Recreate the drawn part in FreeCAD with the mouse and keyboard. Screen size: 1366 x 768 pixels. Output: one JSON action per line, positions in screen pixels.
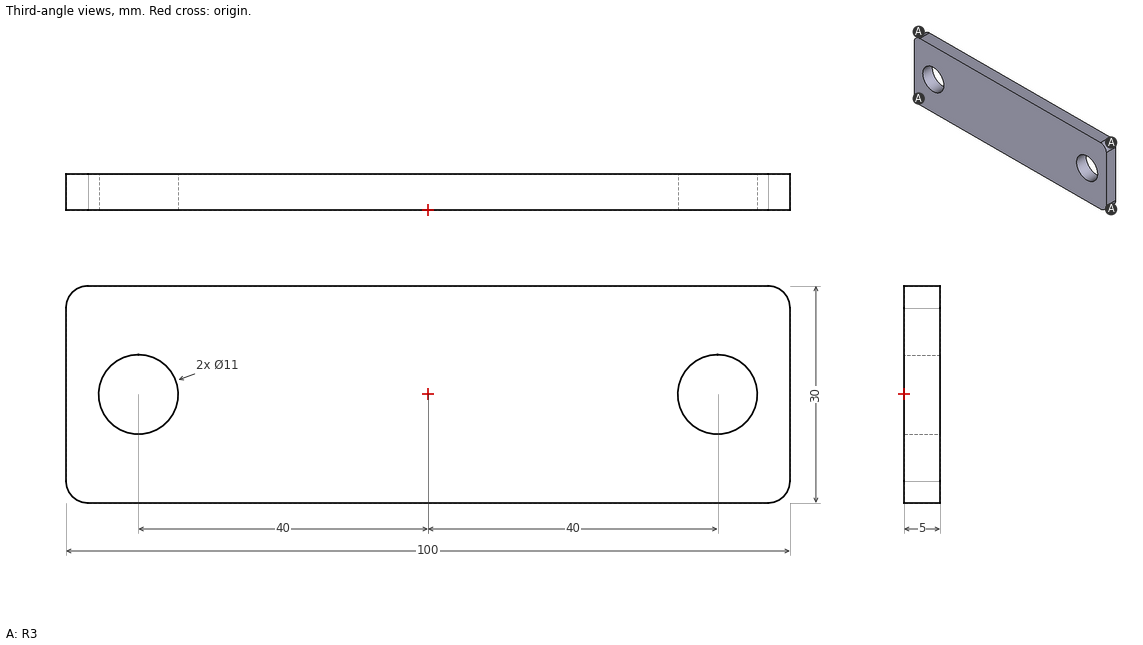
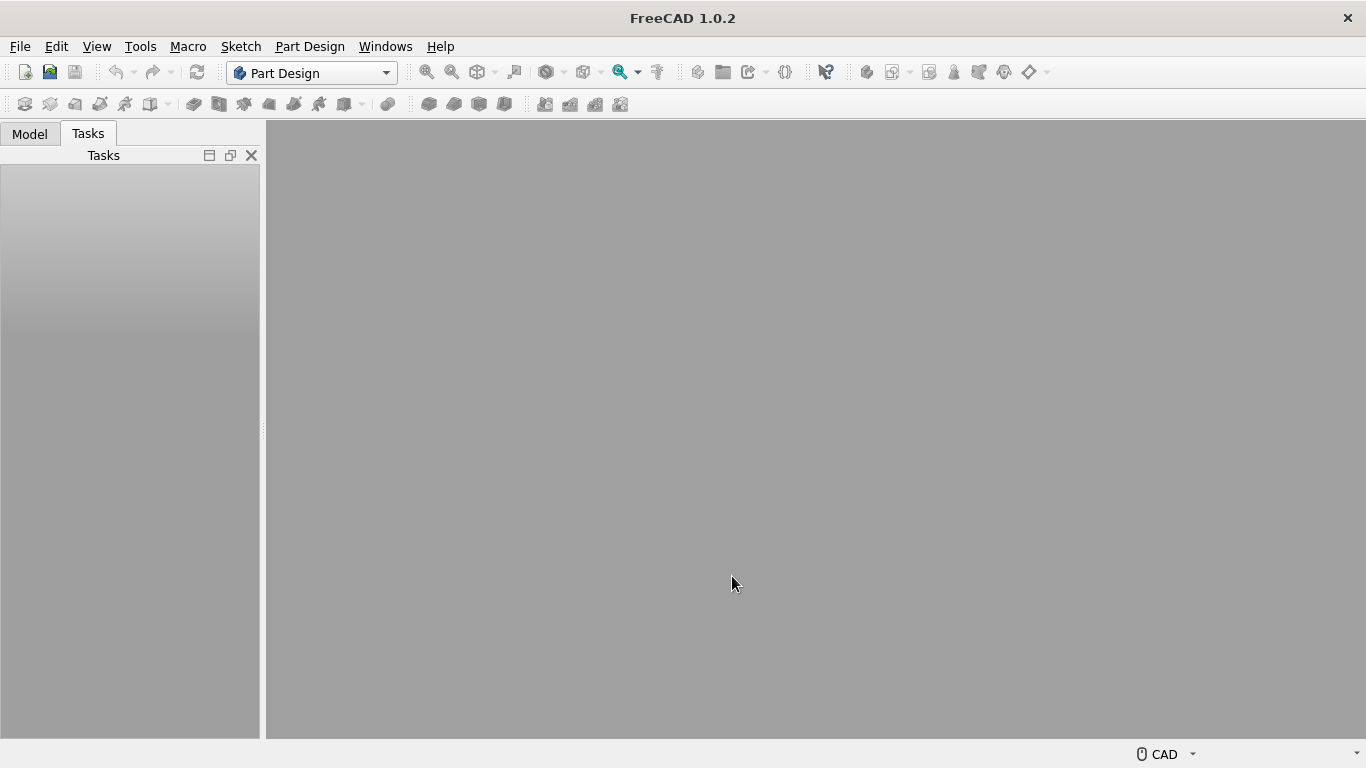
{"action": "key", "text": "ctrl+n"}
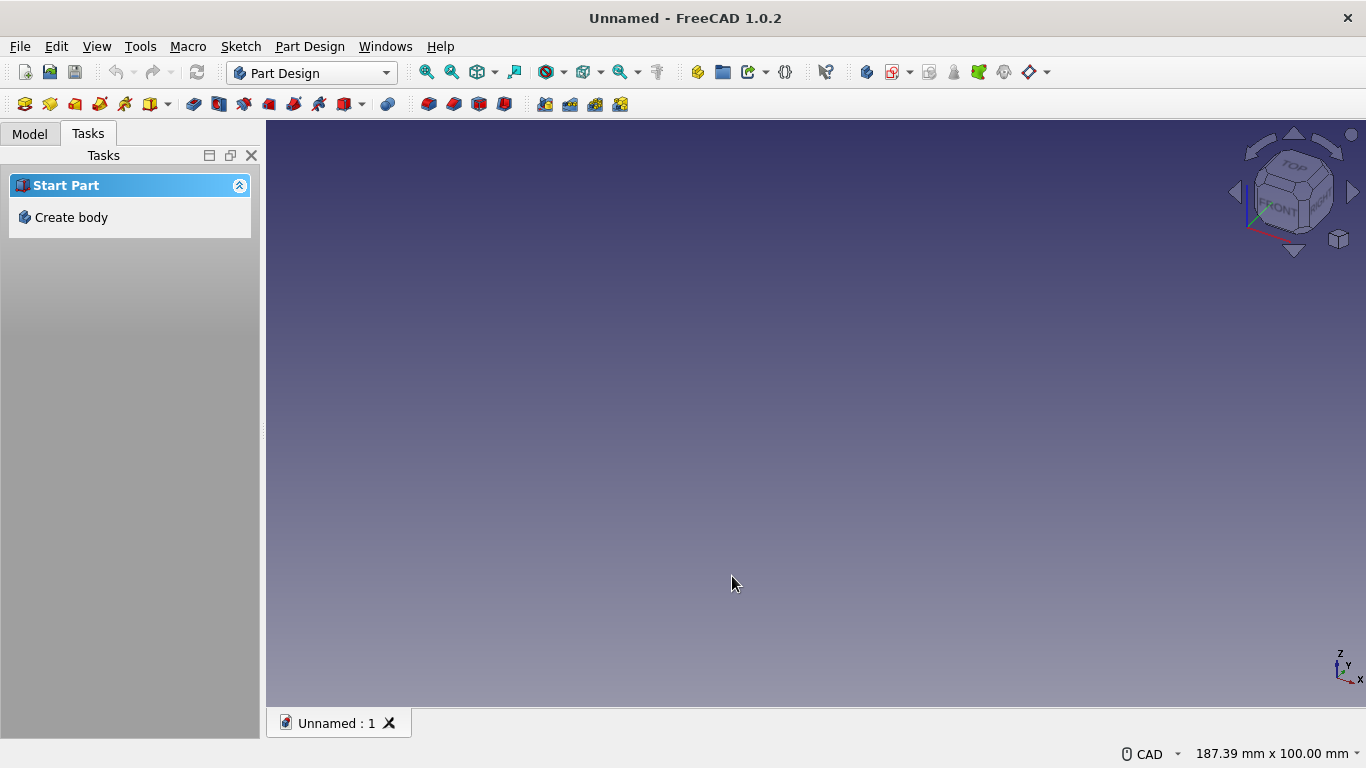
{"action": "left_click", "coordinate": [892, 72]}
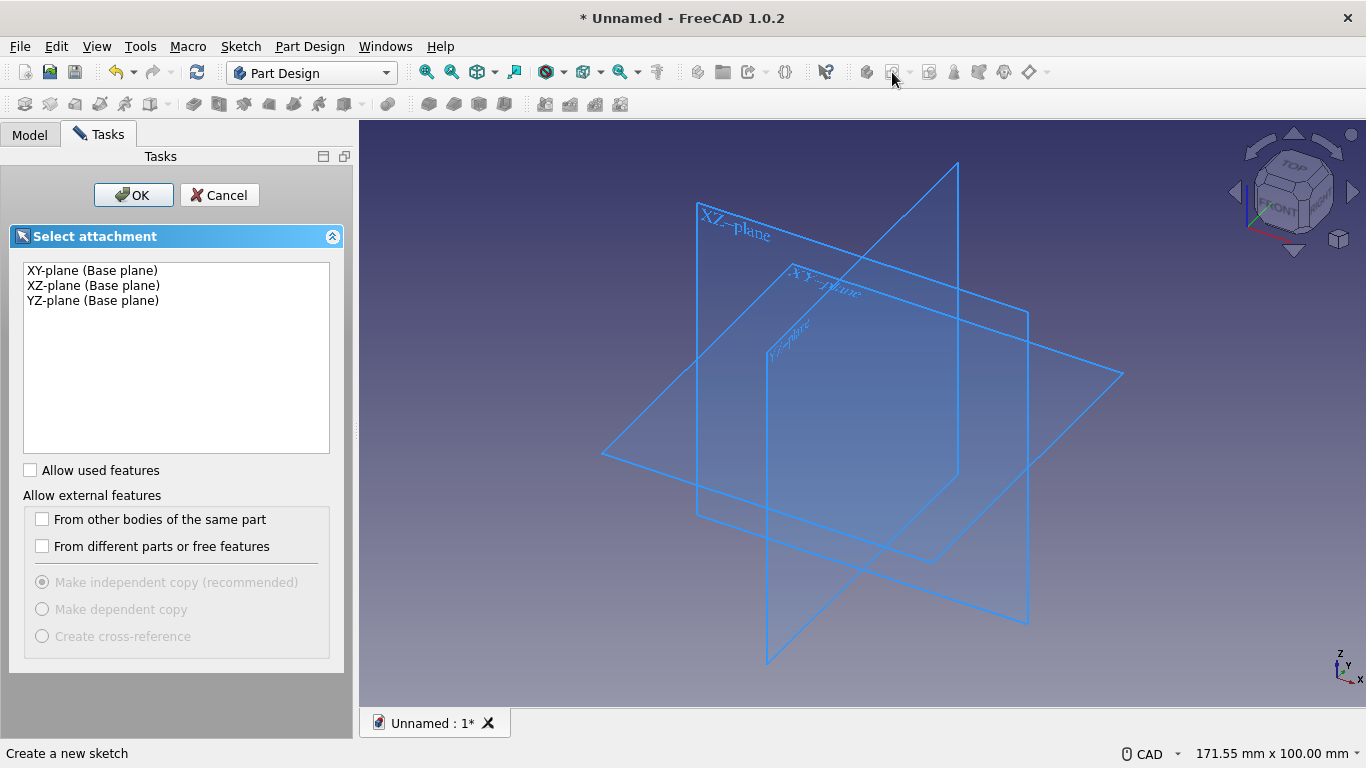
{"action": "left_click", "coordinate": [84, 286]}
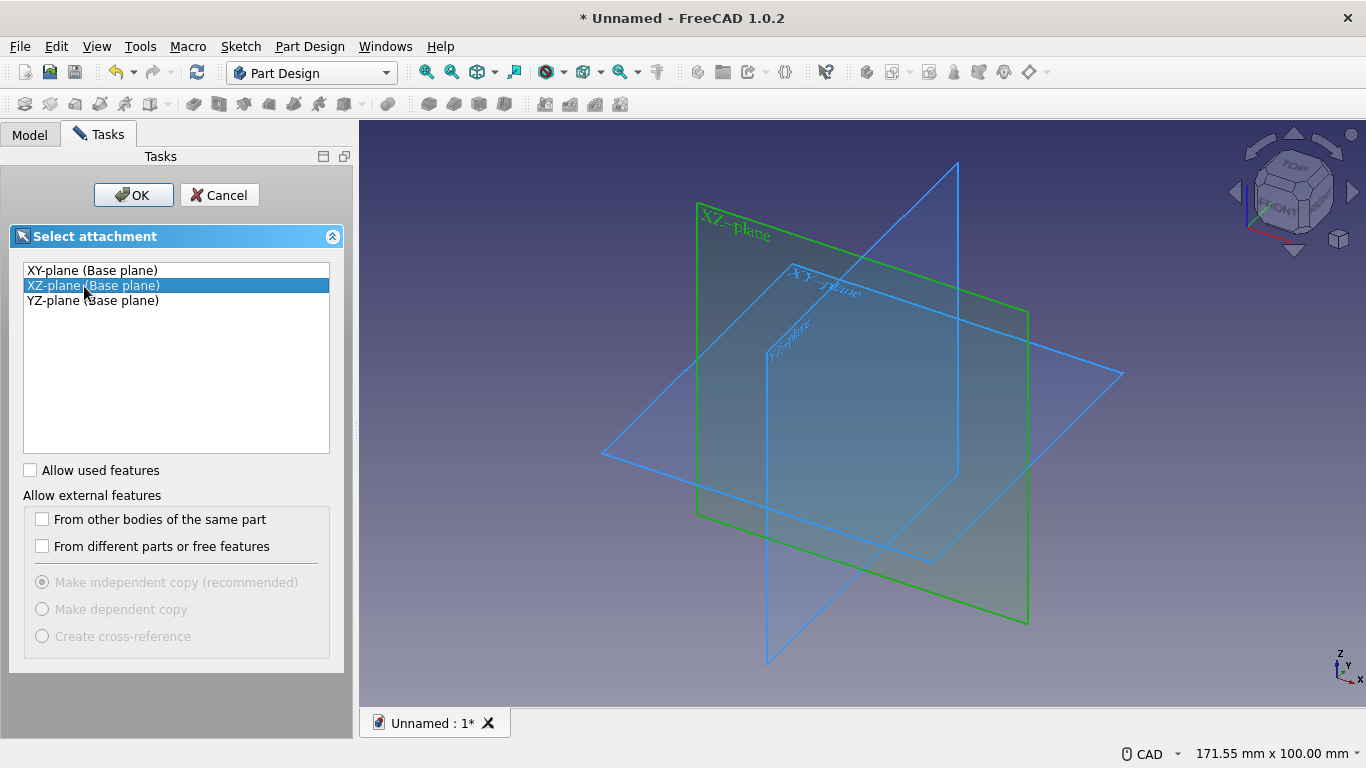
{"action": "left_click", "coordinate": [134, 195]}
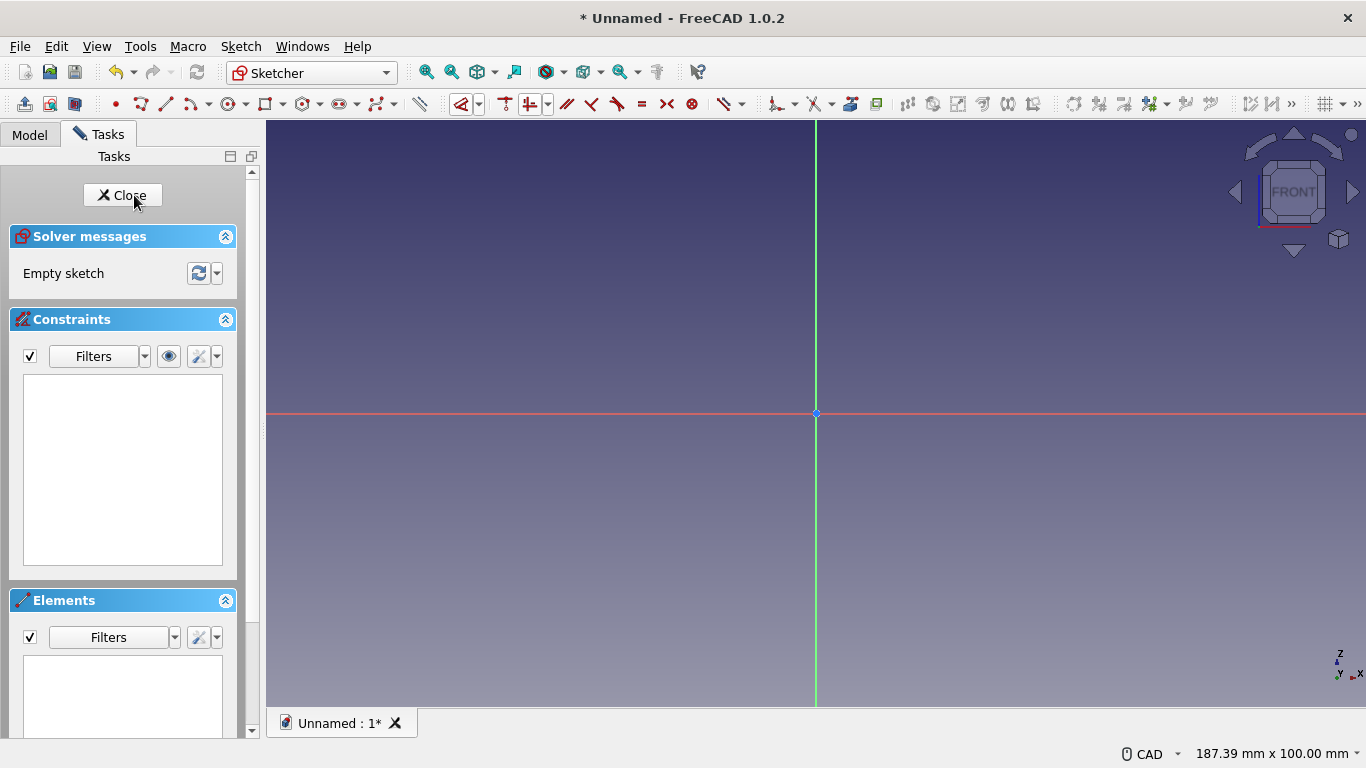
{"action": "key", "text": "g v"}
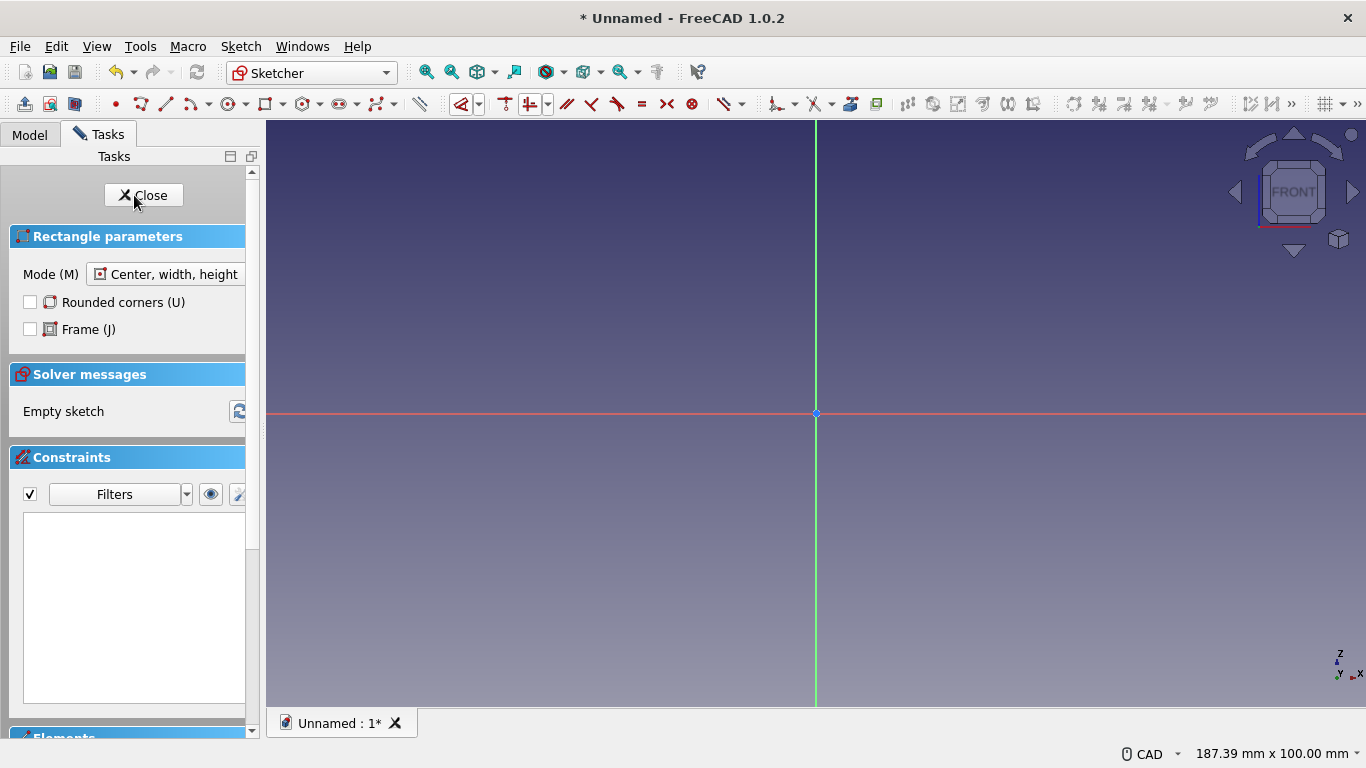
{"action": "left_click", "coordinate": [816, 414]}
{"action": "mouse_move", "coordinate": [1110, 325]}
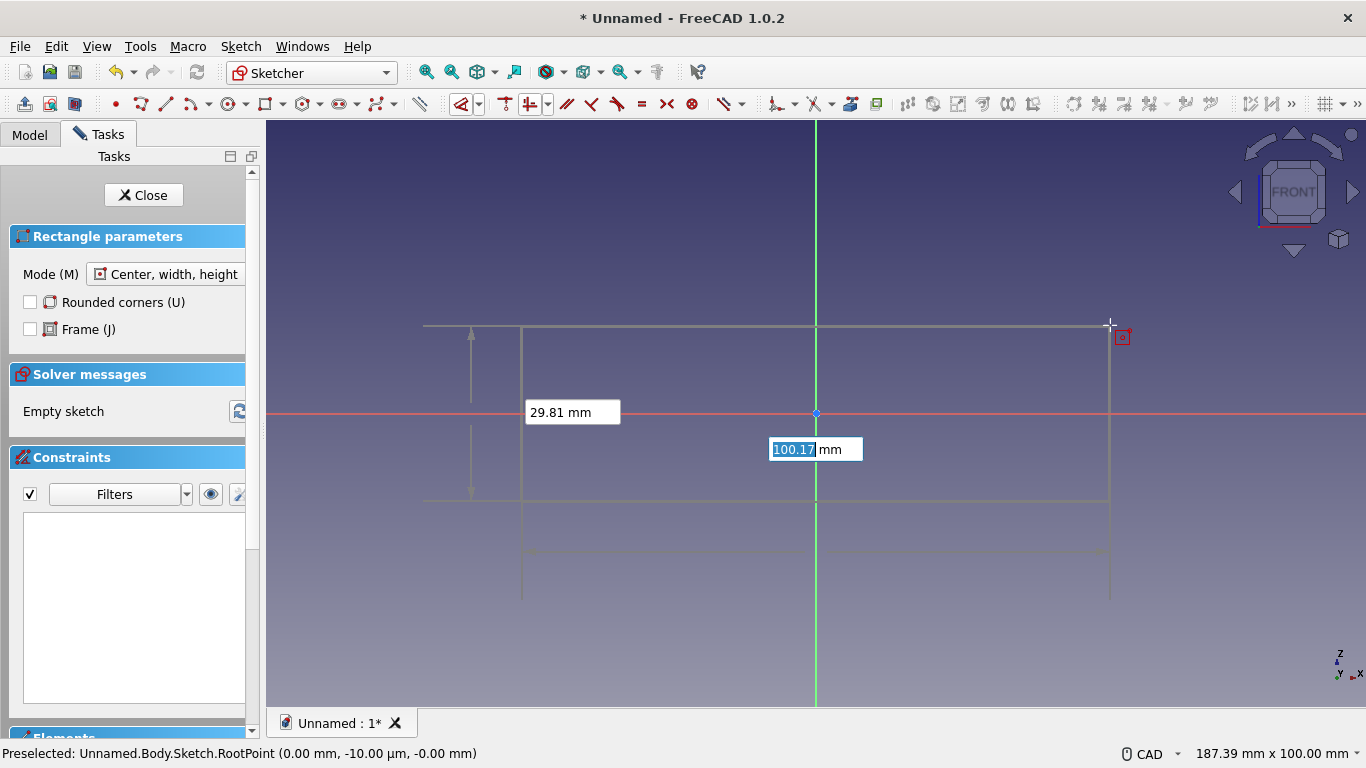
{"action": "type", "text": "100"}
{"action": "key", "text": "Tab"}
{"action": "type", "text": "30"}
{"action": "key", "text": "Return"}
{"action": "key", "text": "Escape"}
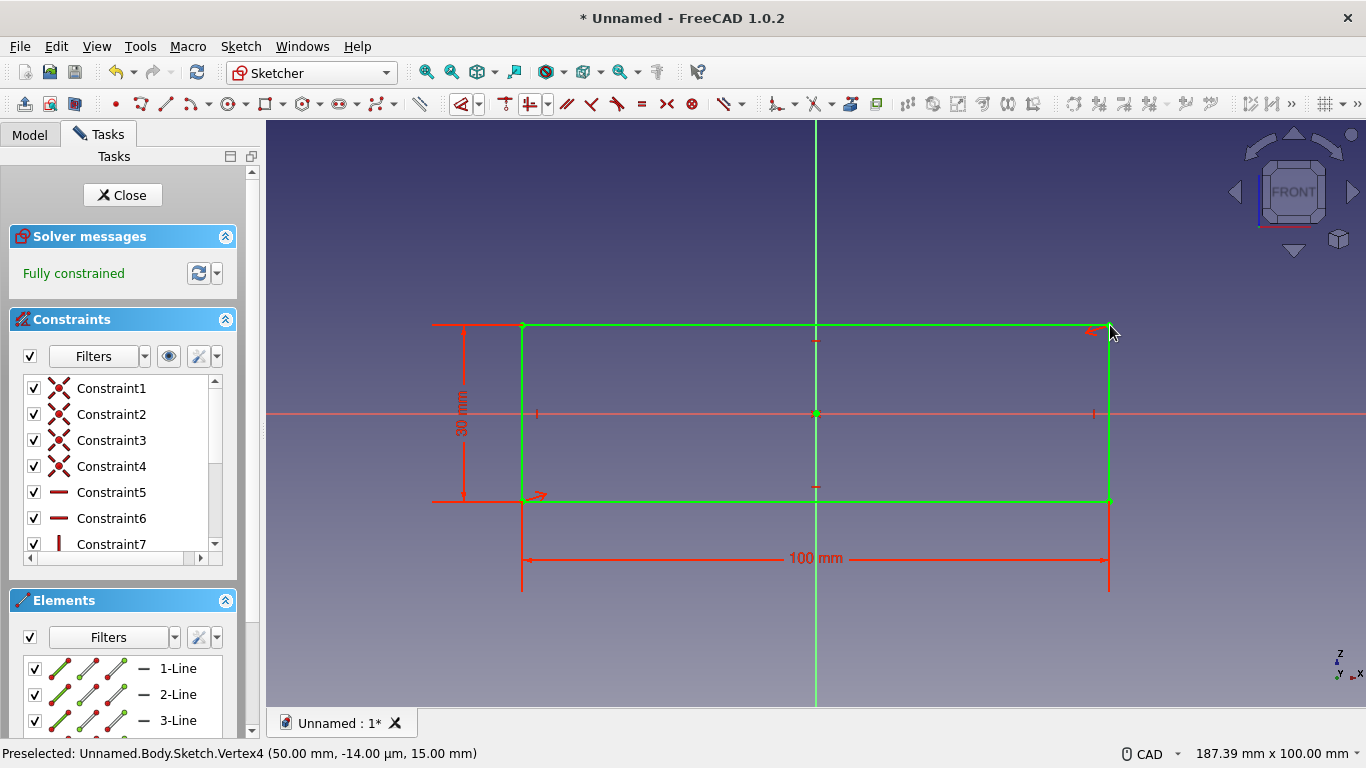
{"action": "left_click", "coordinate": [123, 195]}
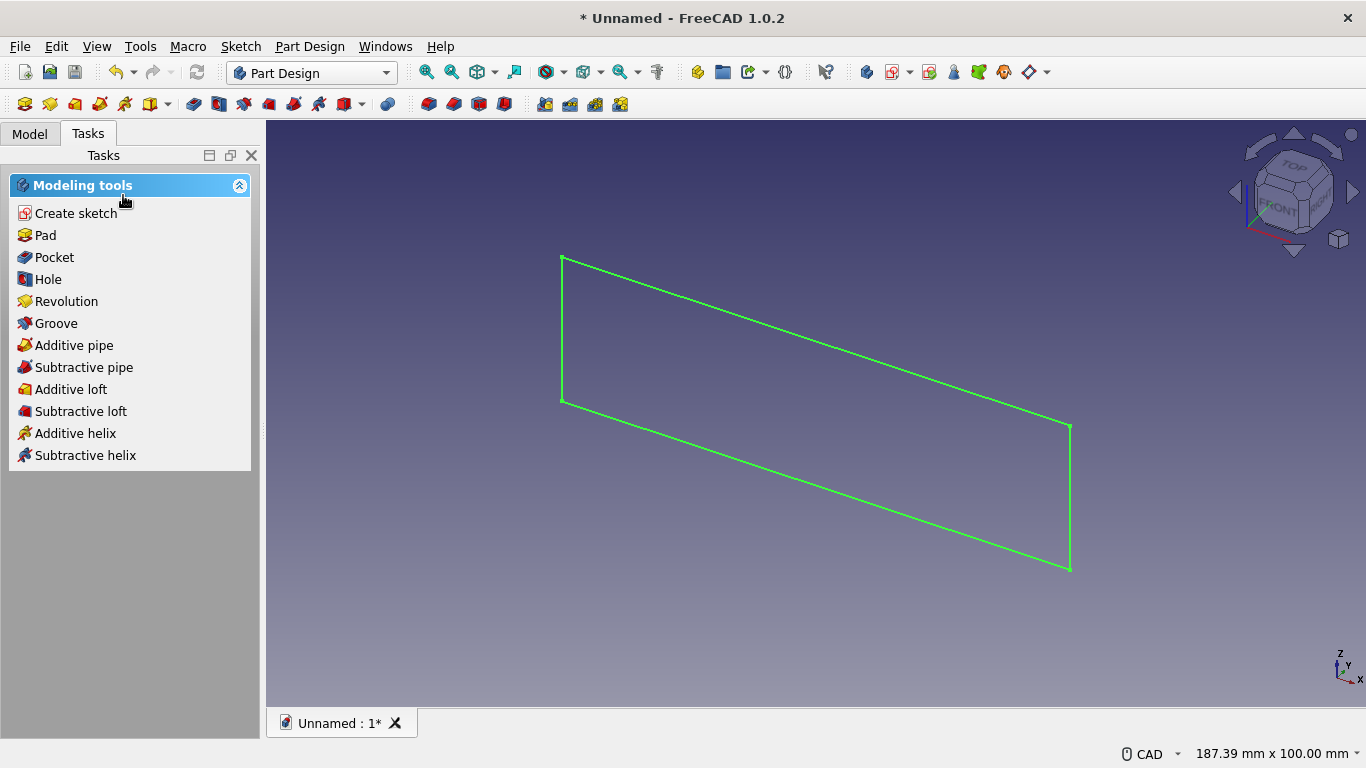
{"action": "left_click", "coordinate": [25, 104]}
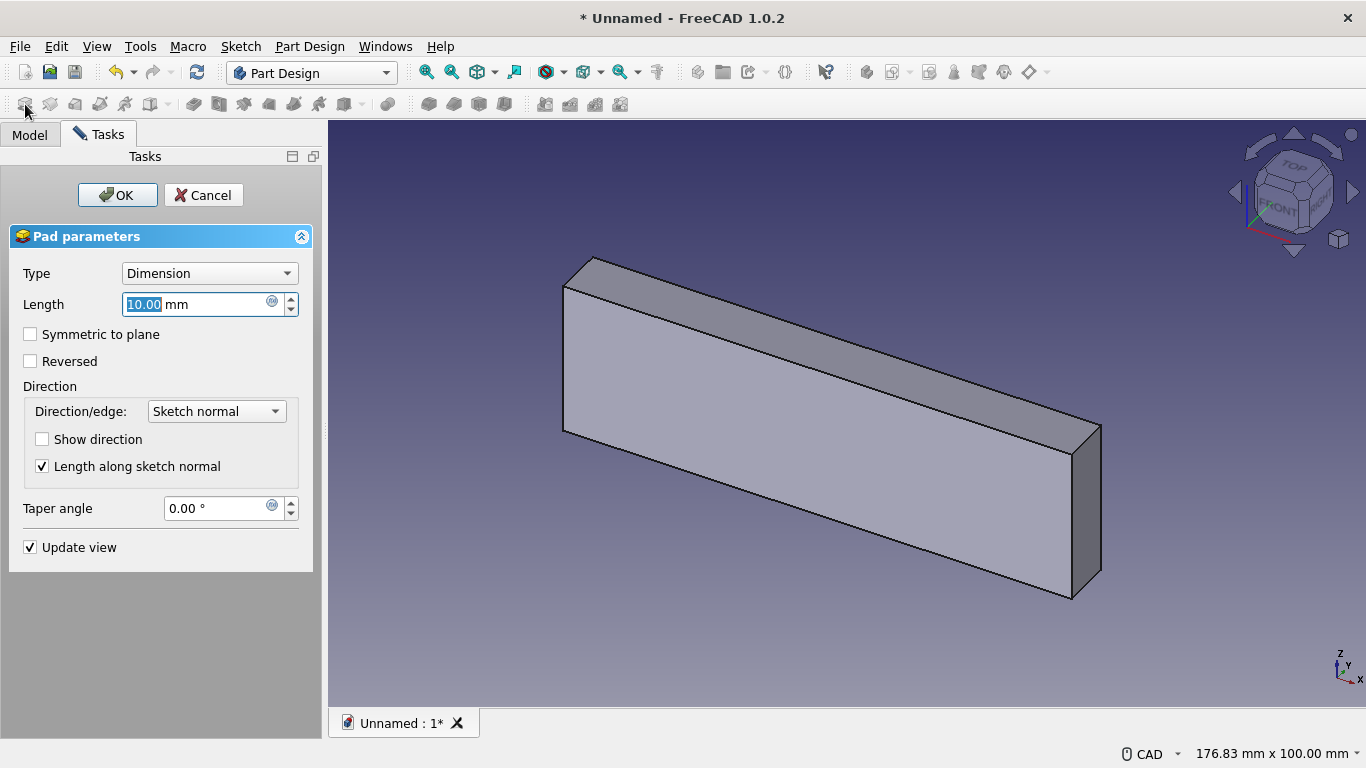
{"action": "type", "text": "5"}
{"action": "key", "text": "Tab"}